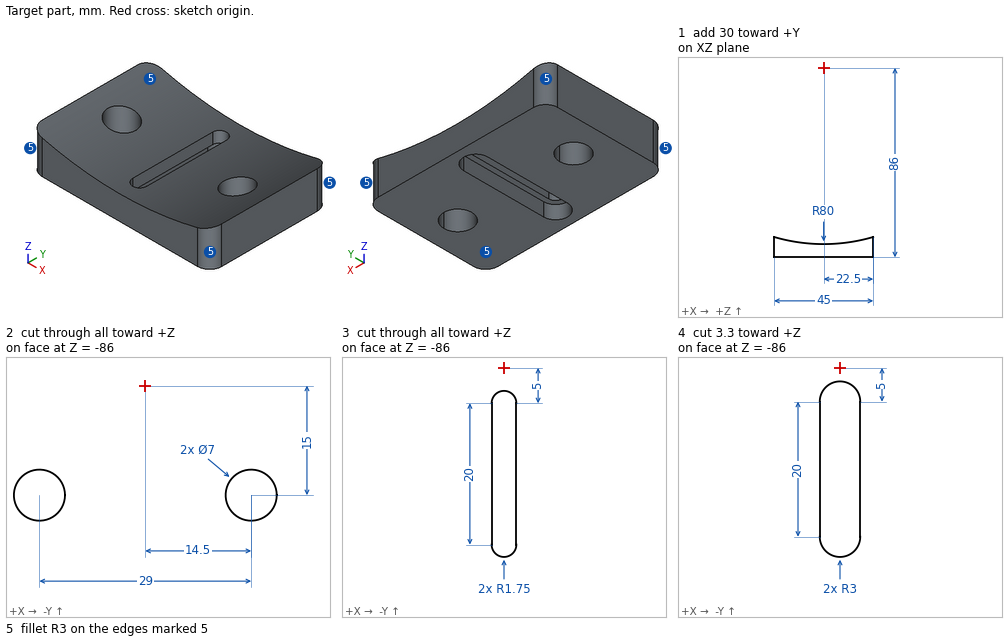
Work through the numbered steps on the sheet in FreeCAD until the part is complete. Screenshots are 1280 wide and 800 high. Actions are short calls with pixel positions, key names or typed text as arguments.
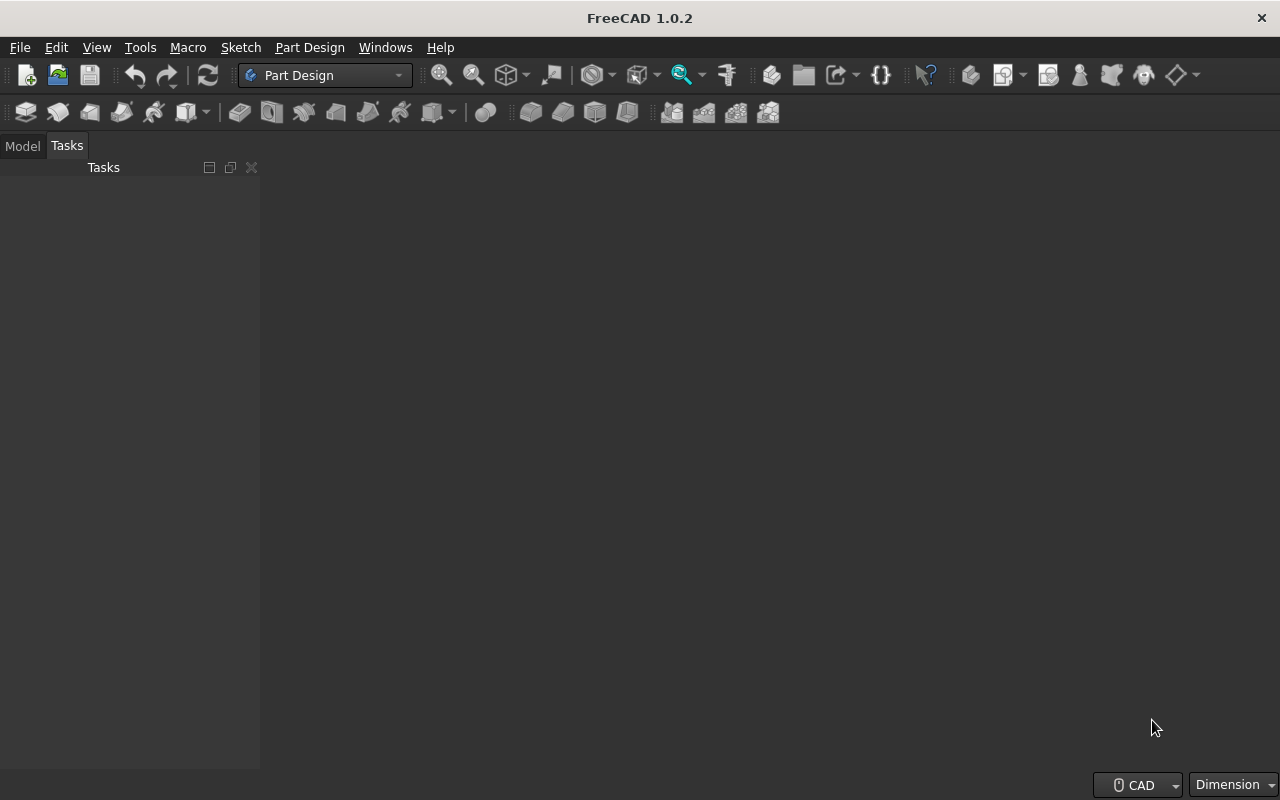
click(26, 76)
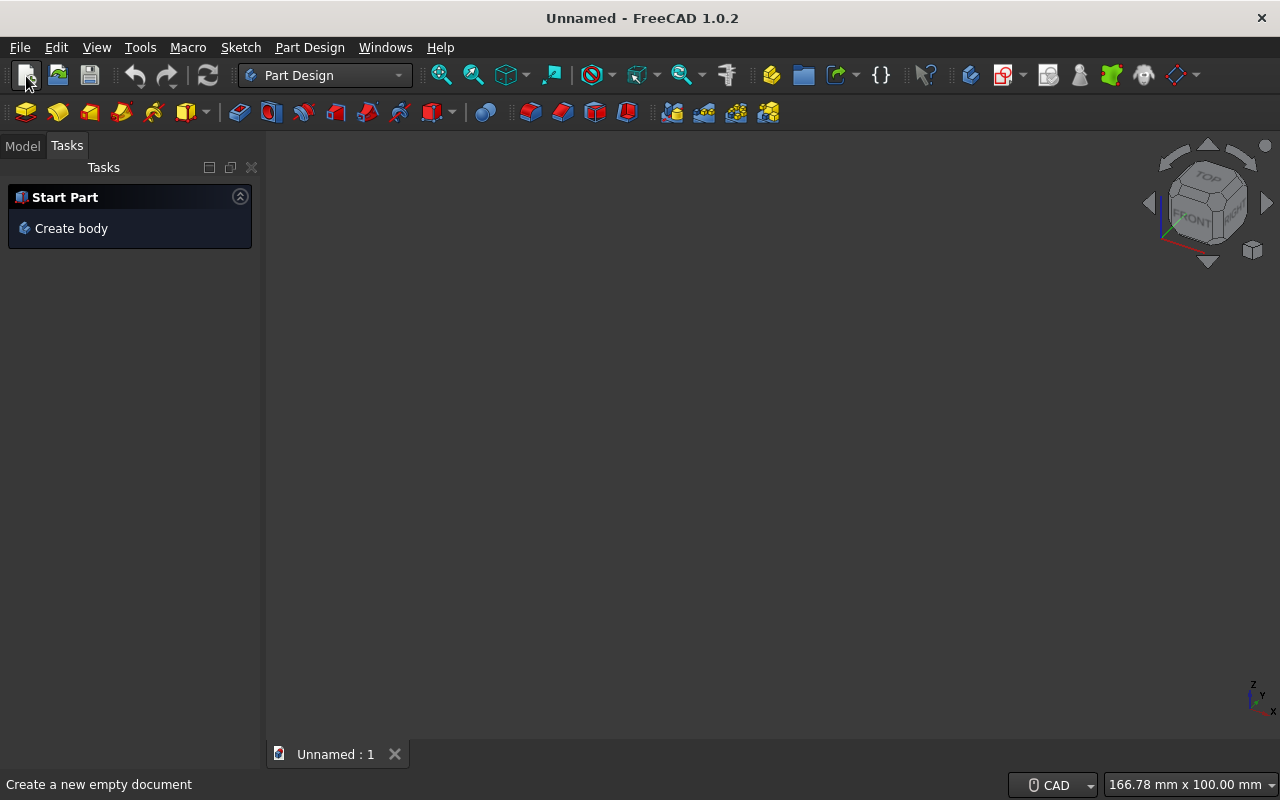
click(1004, 76)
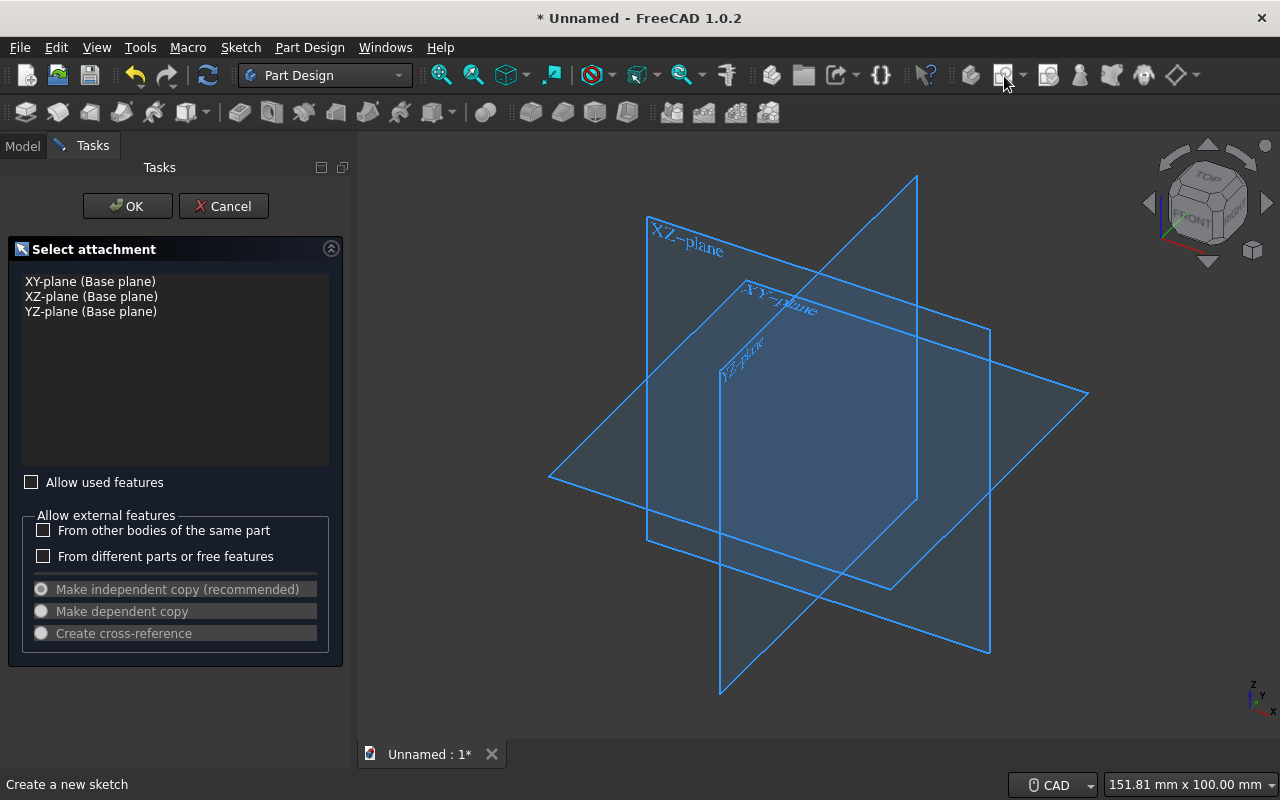
click(82, 296)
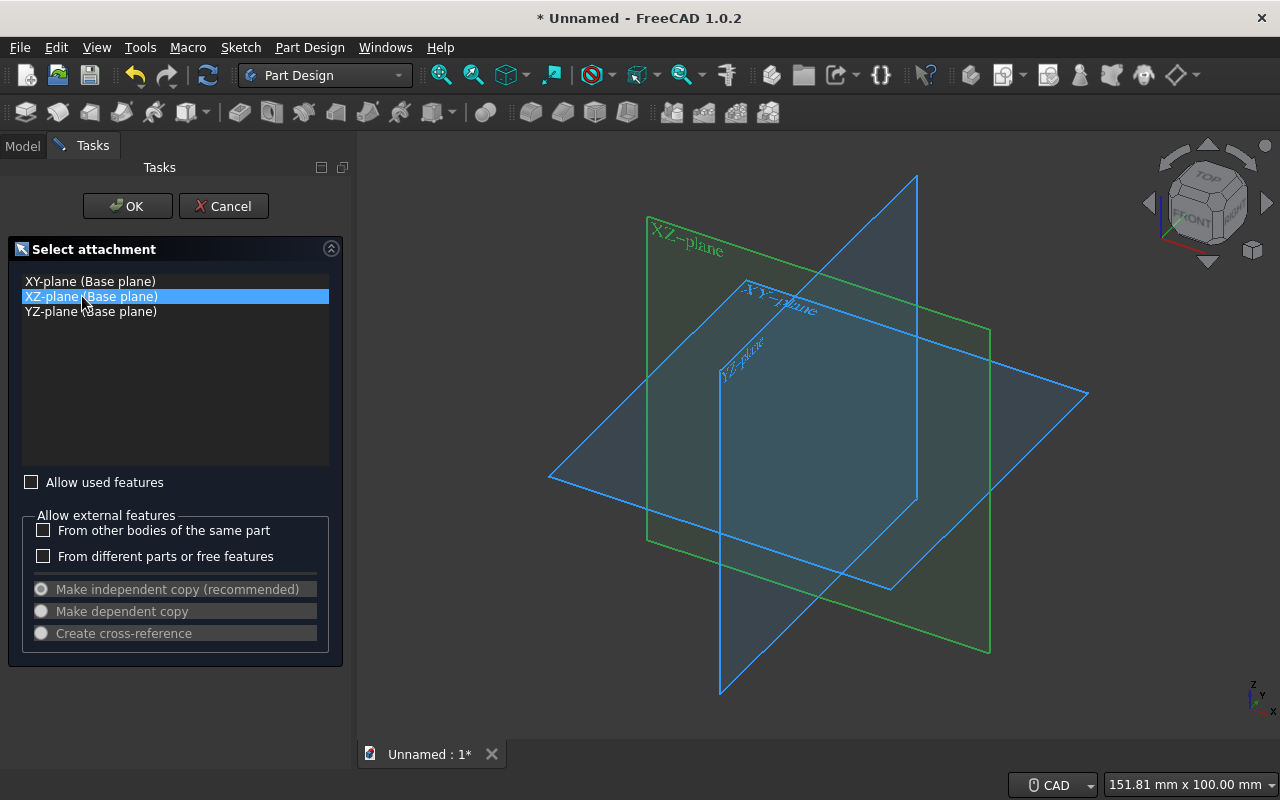
click(128, 206)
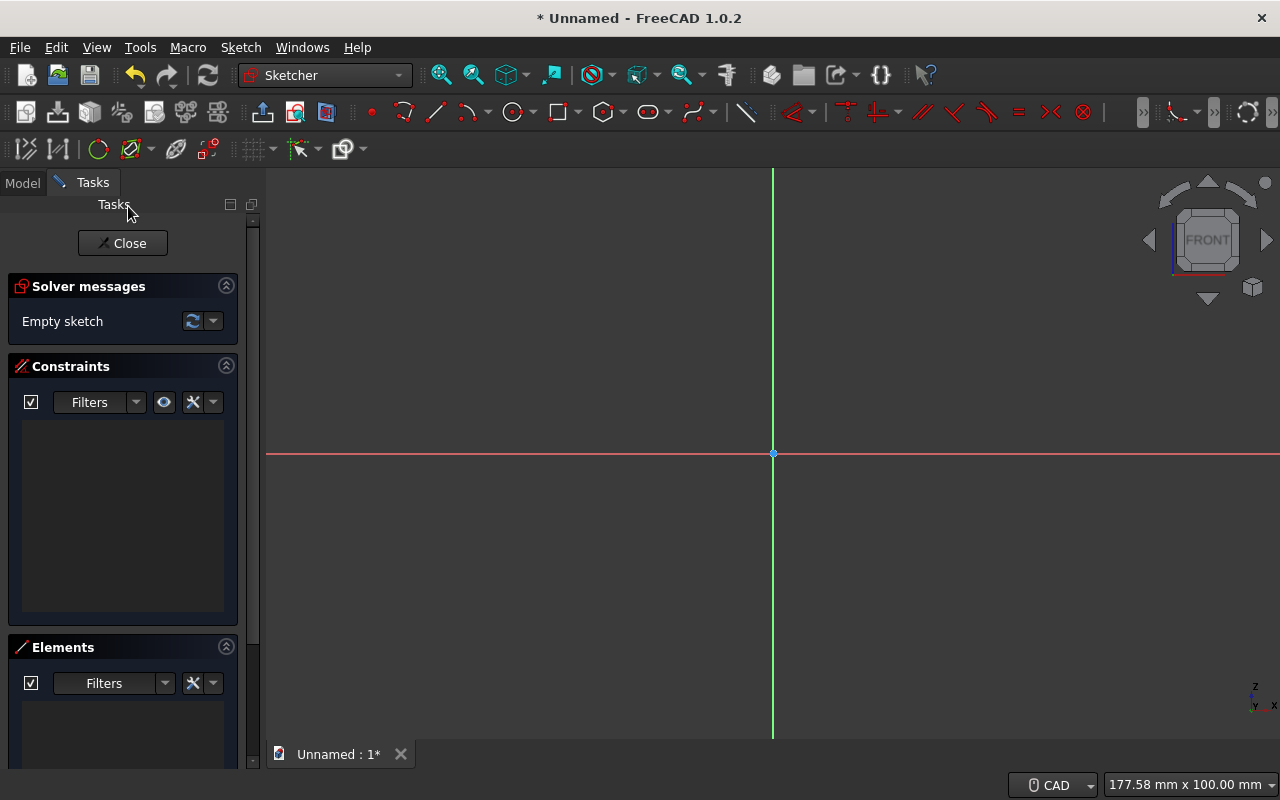
scroll(621, 196, down, 3)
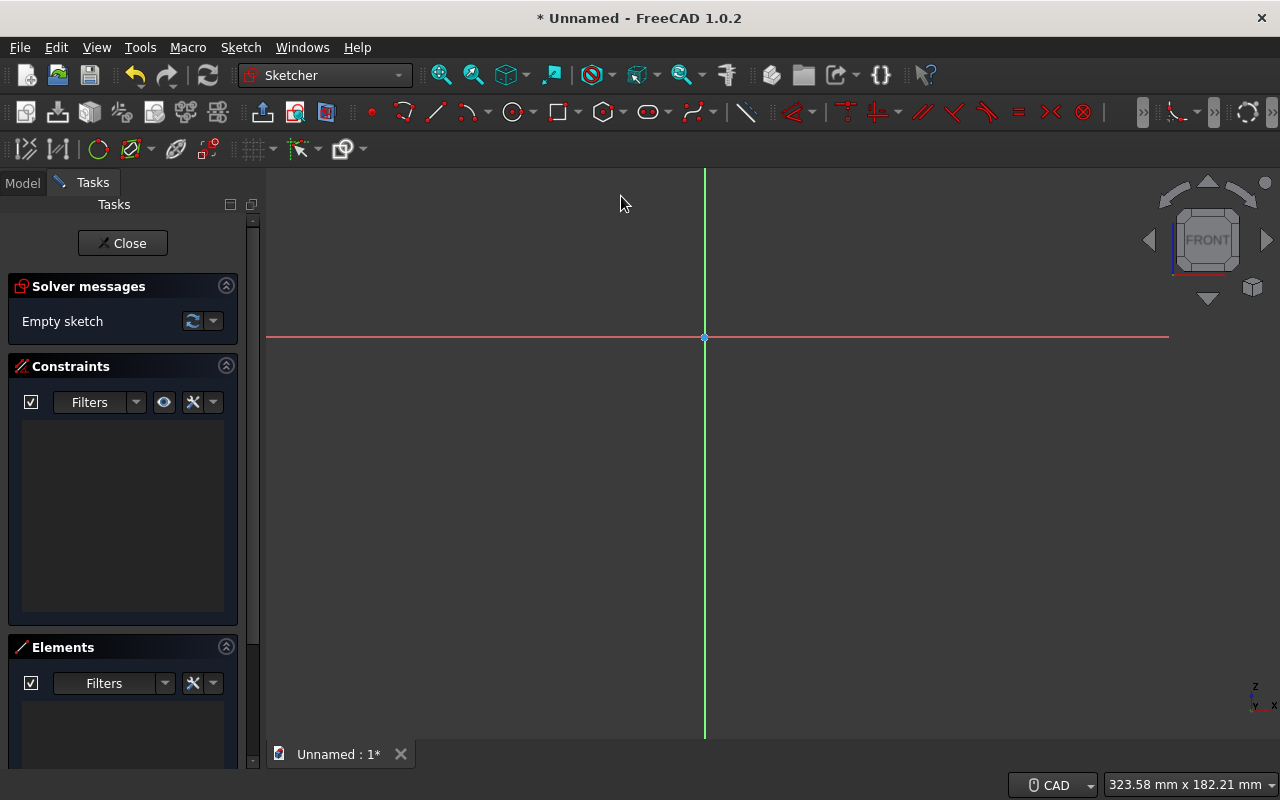
click(404, 112)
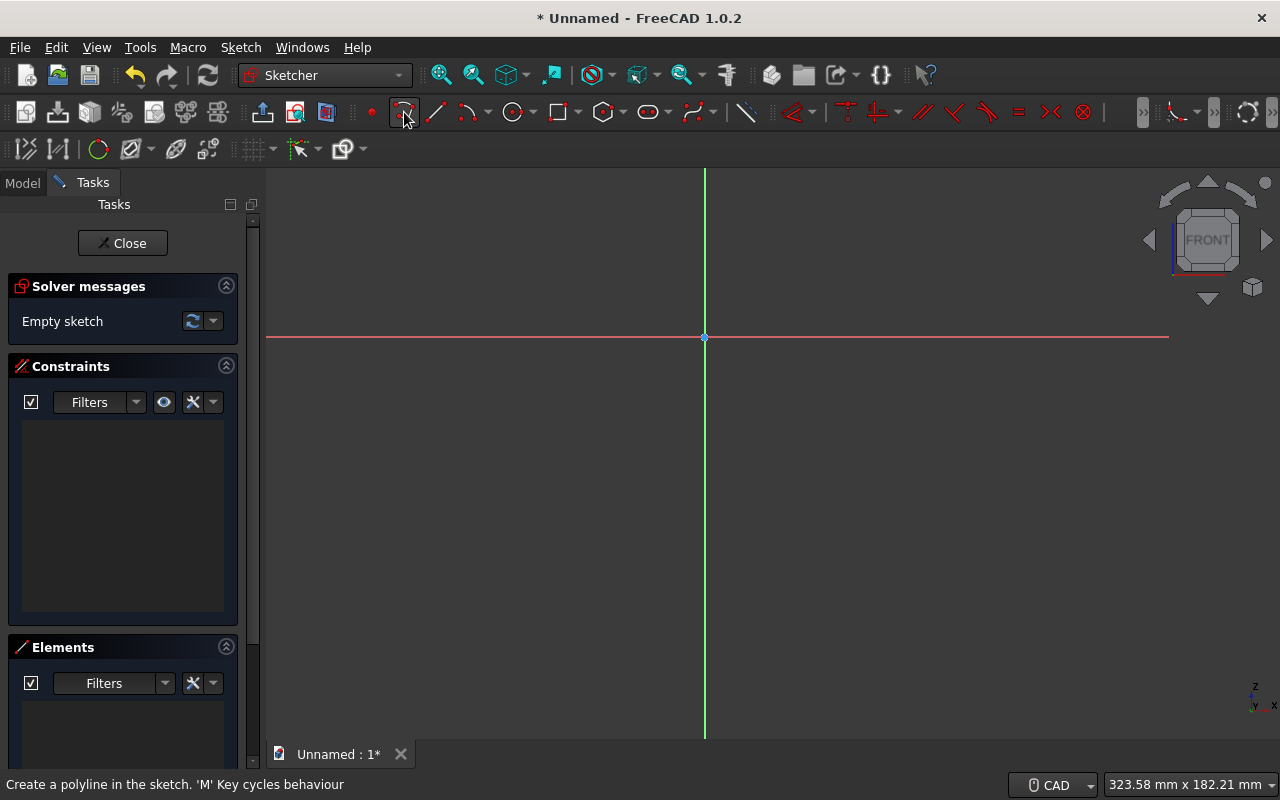
click(775, 578)
click(775, 607)
click(634, 607)
click(634, 578)
right_click(634, 578)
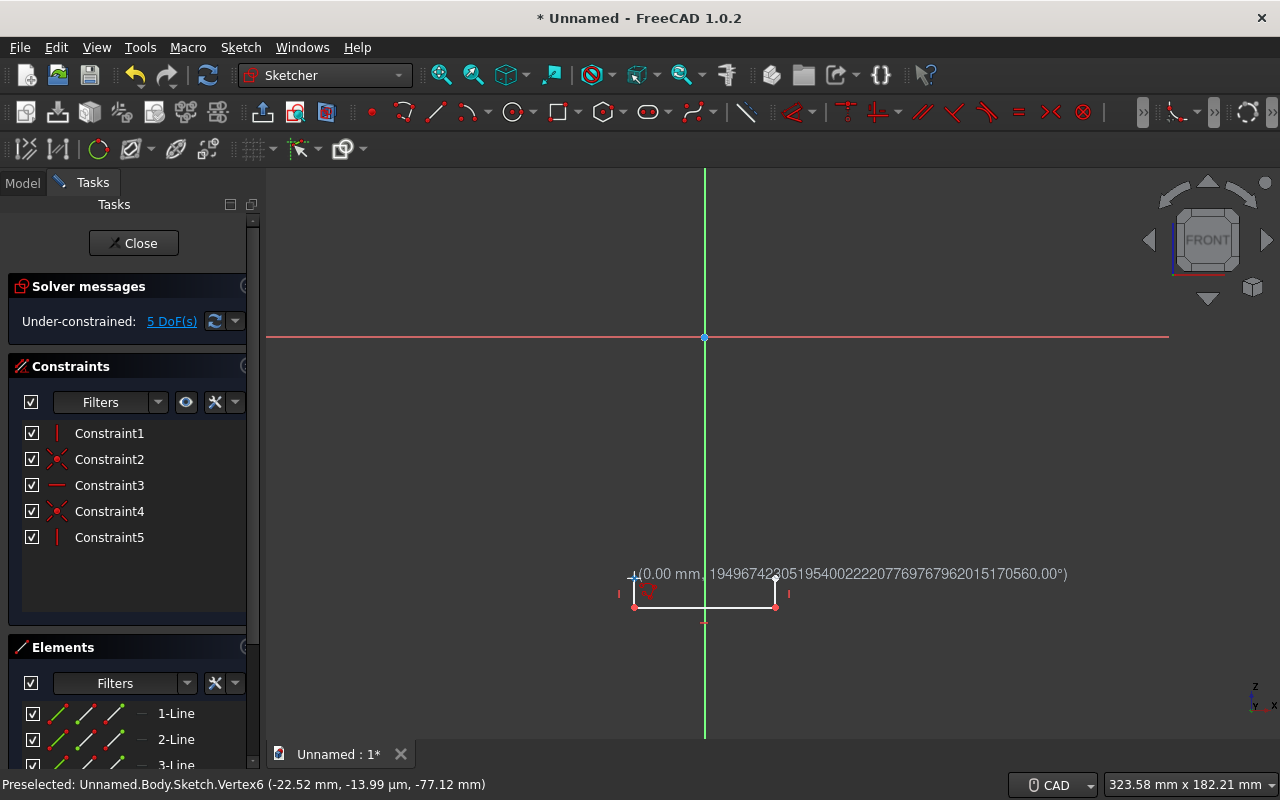
key(g)
key(3)
key(a)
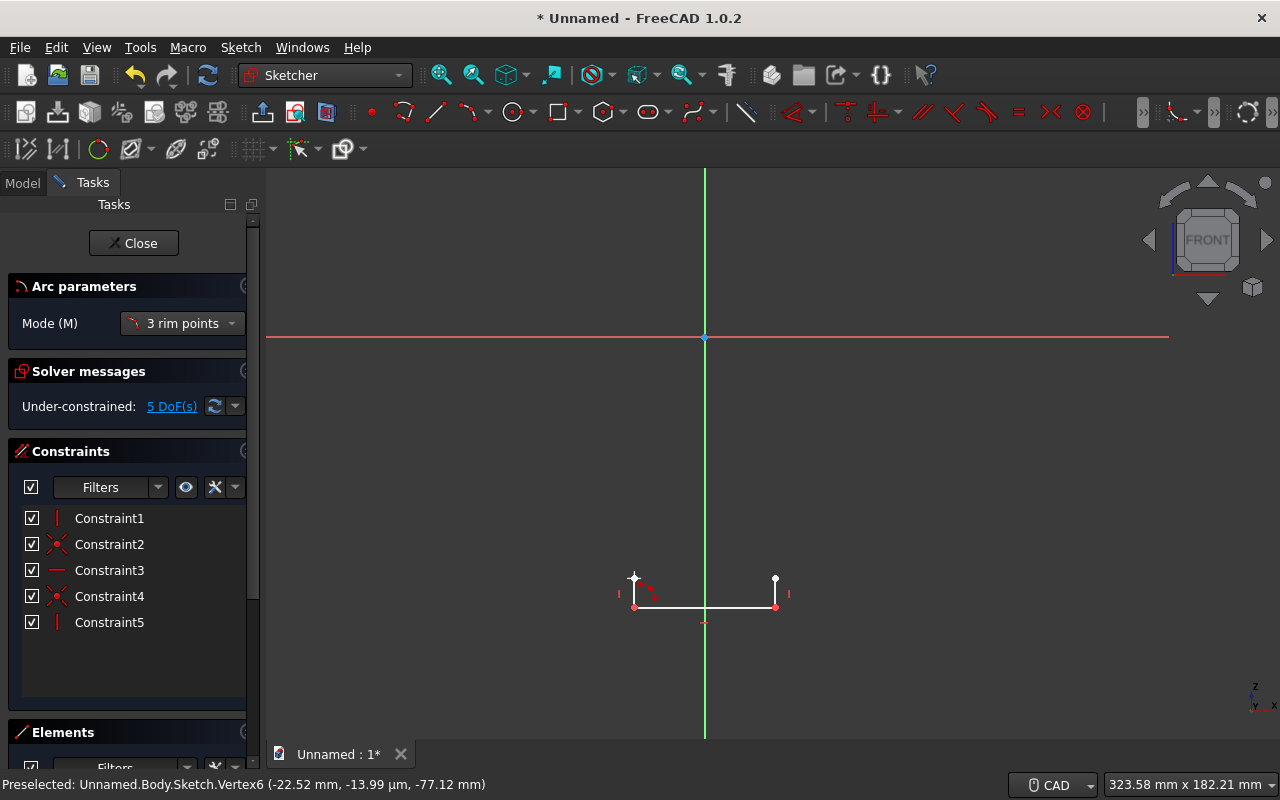
click(634, 579)
click(775, 579)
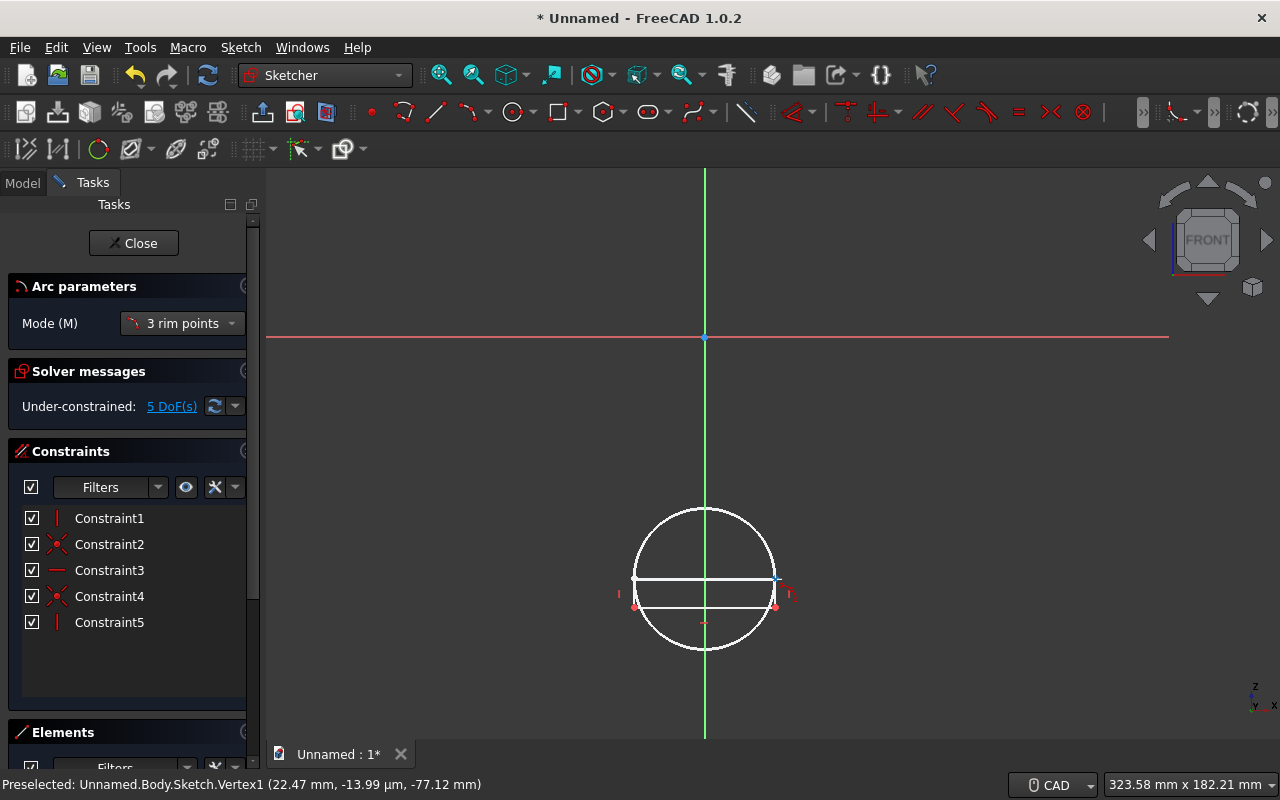
scroll(690, 588, up, 3)